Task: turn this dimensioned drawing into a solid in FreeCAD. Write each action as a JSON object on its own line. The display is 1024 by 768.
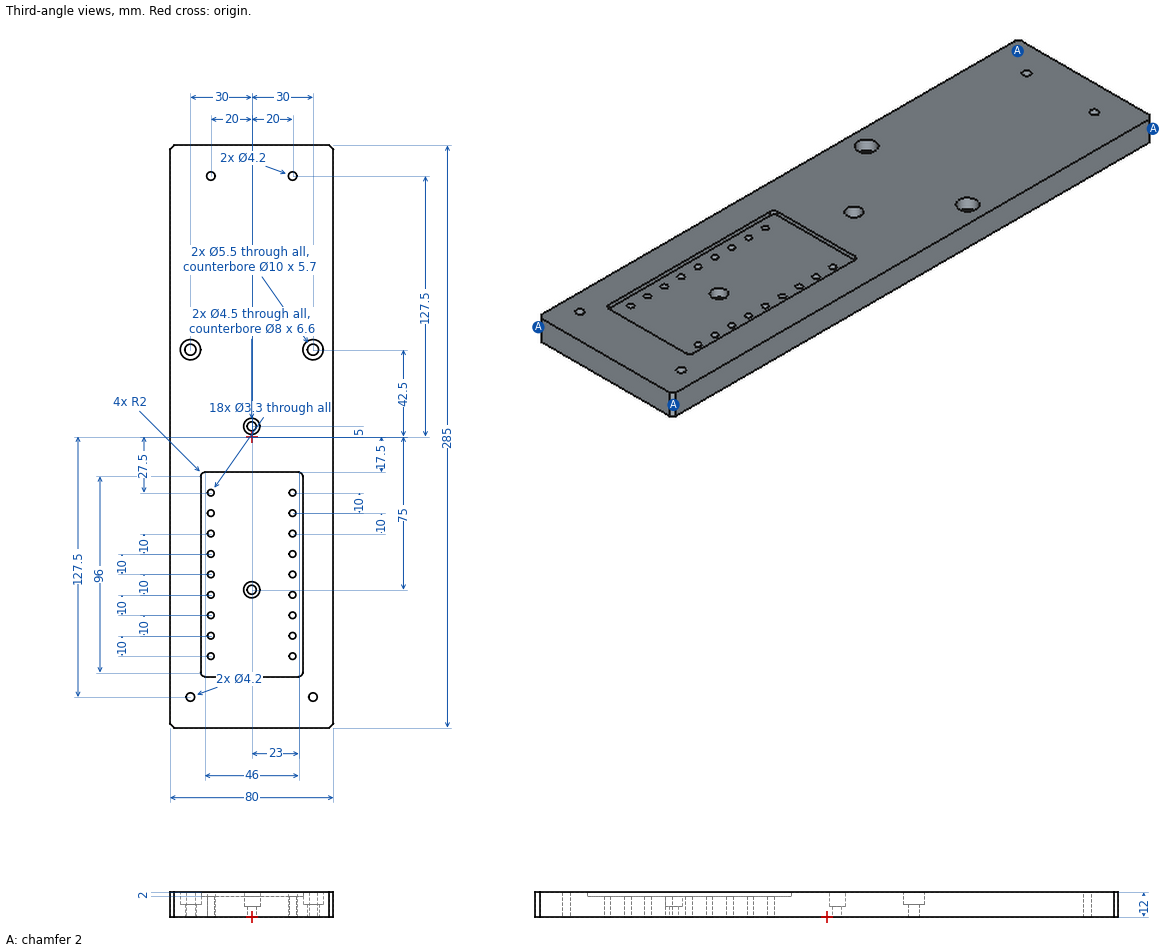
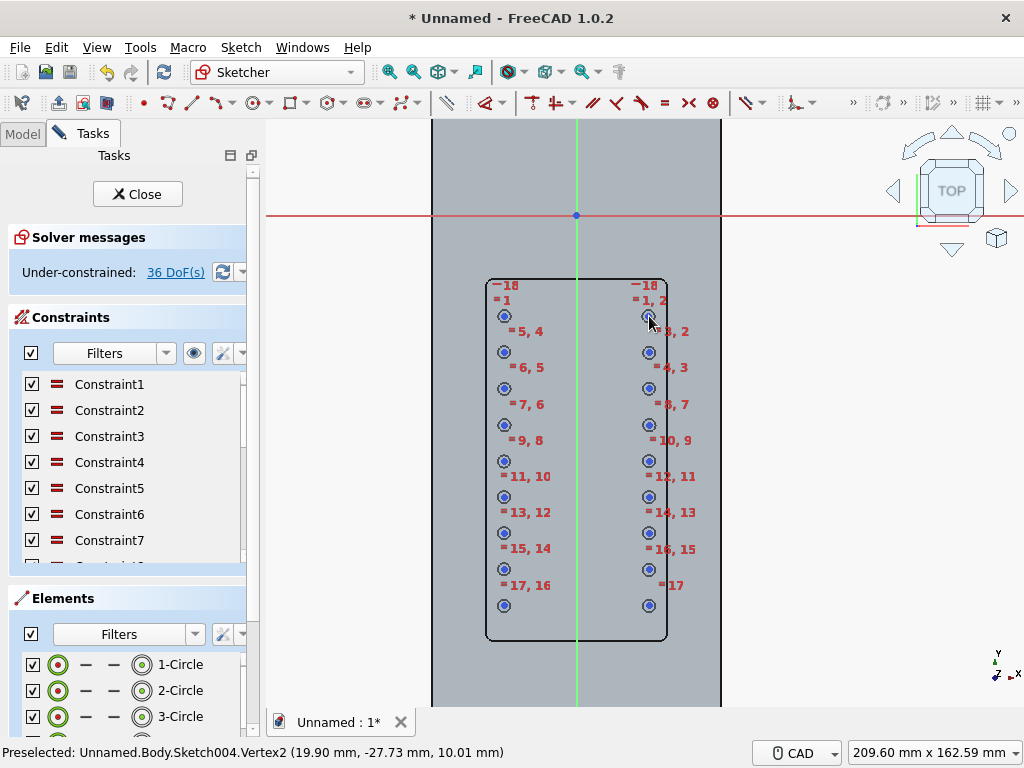
{"action": "left_click", "coordinate": [649, 316]}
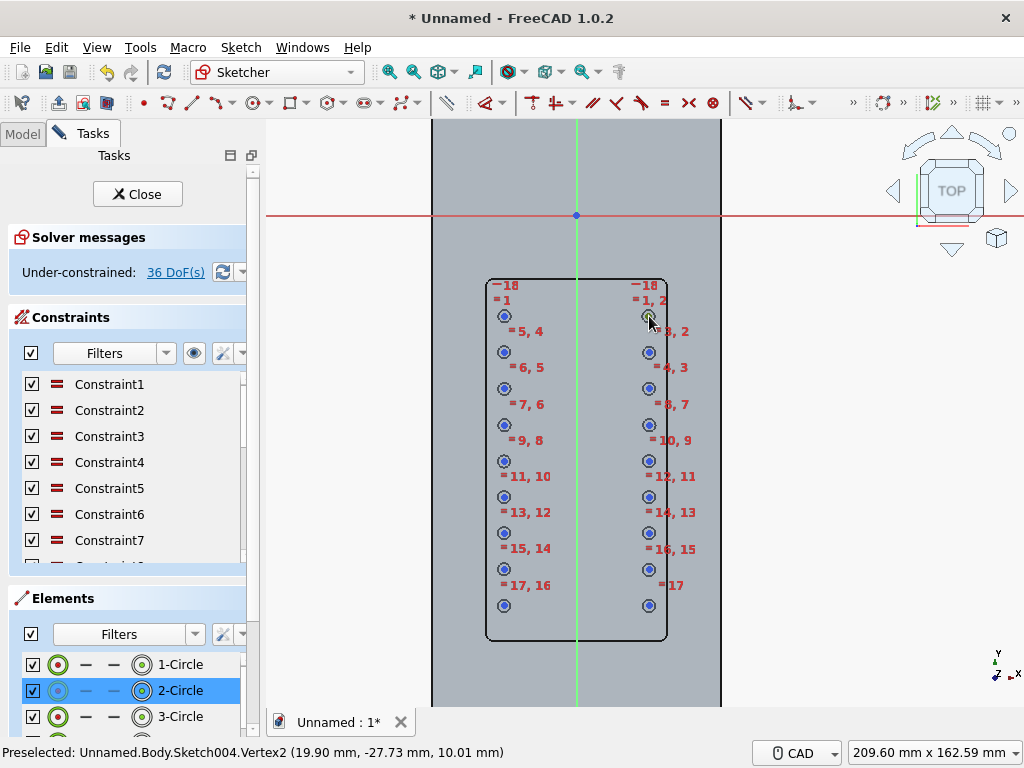
{"action": "left_click", "coordinate": [649, 353]}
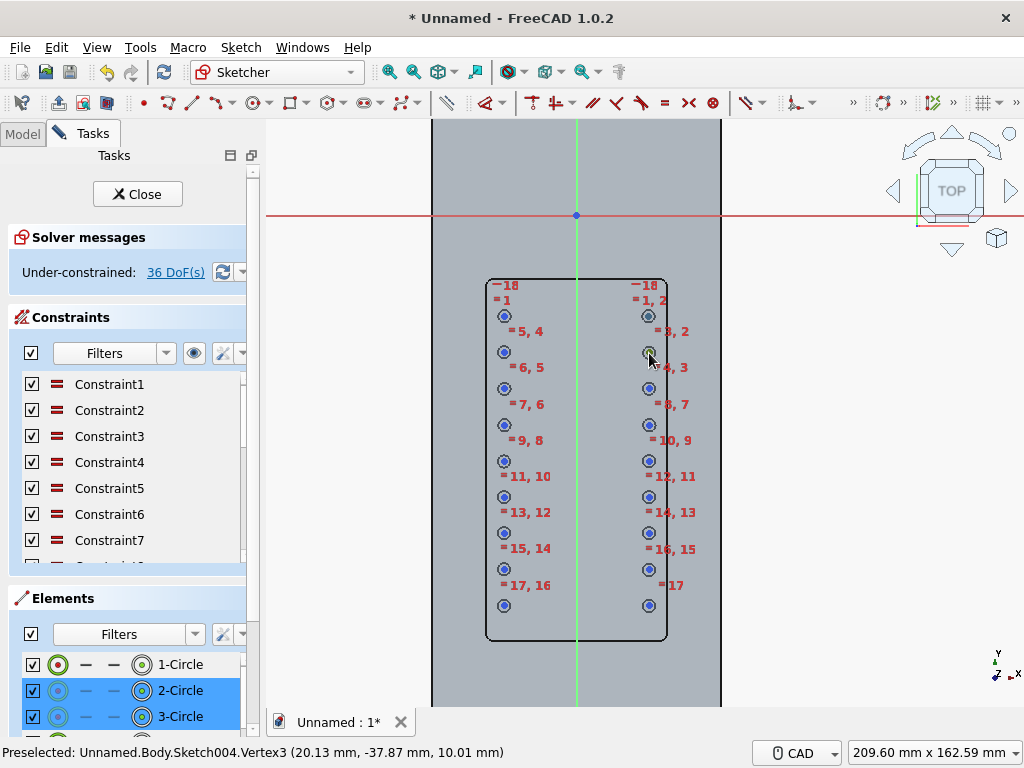
{"action": "key", "text": "v"}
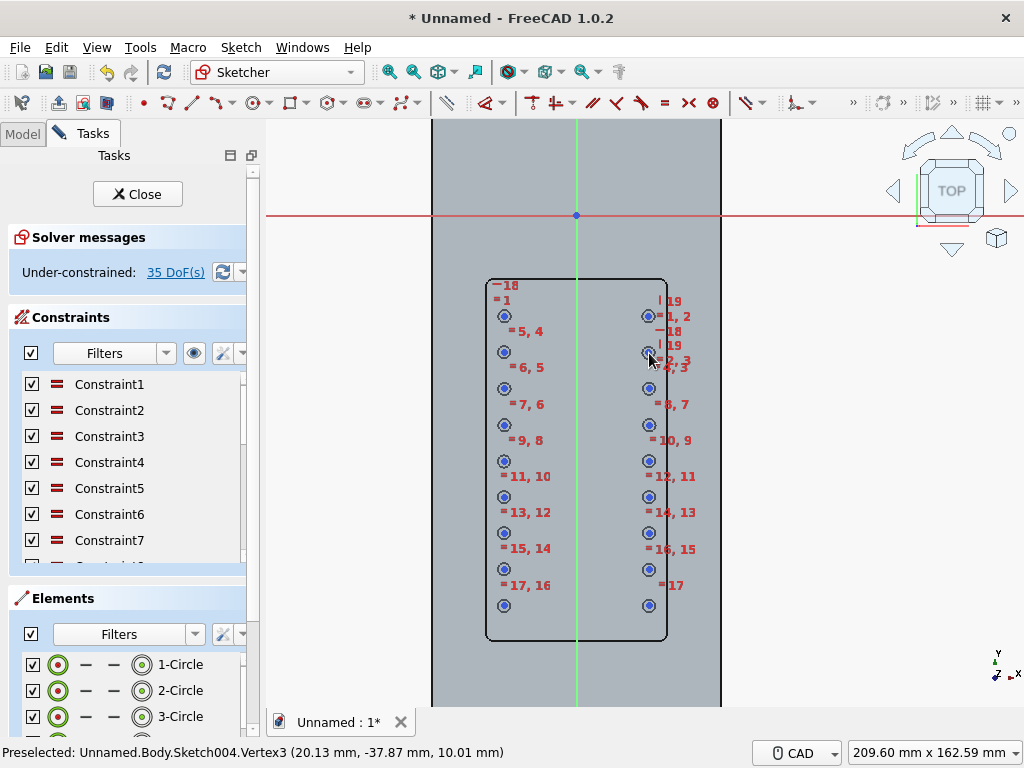
{"action": "left_click", "coordinate": [649, 353]}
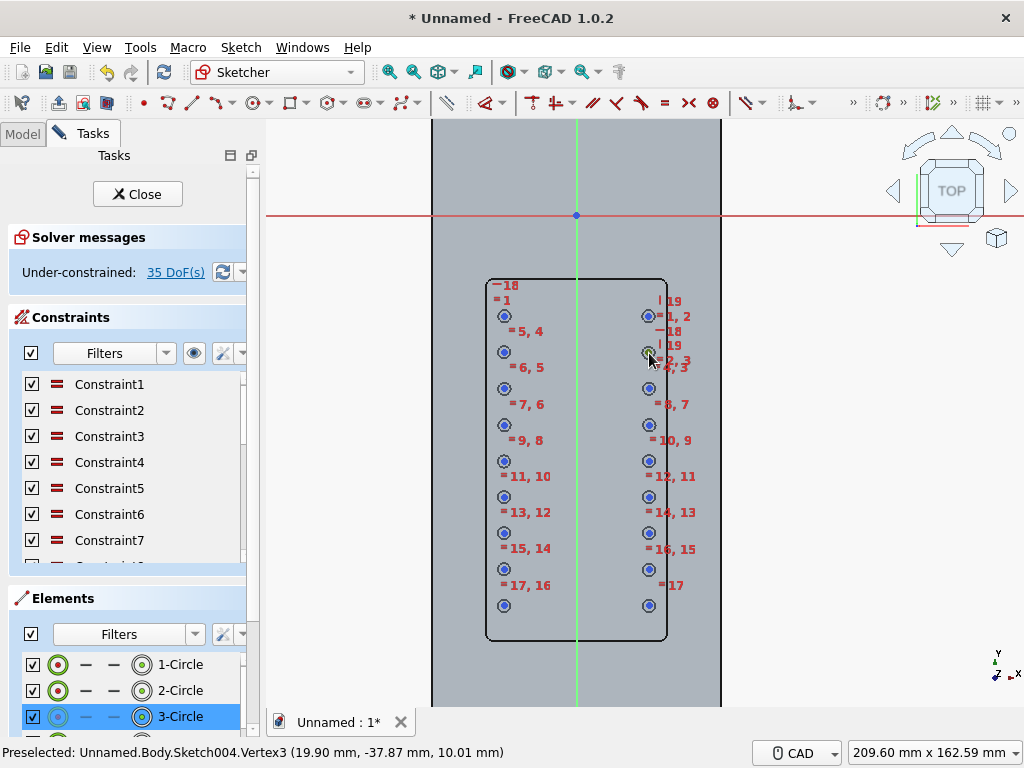
{"action": "left_click", "coordinate": [649, 389]}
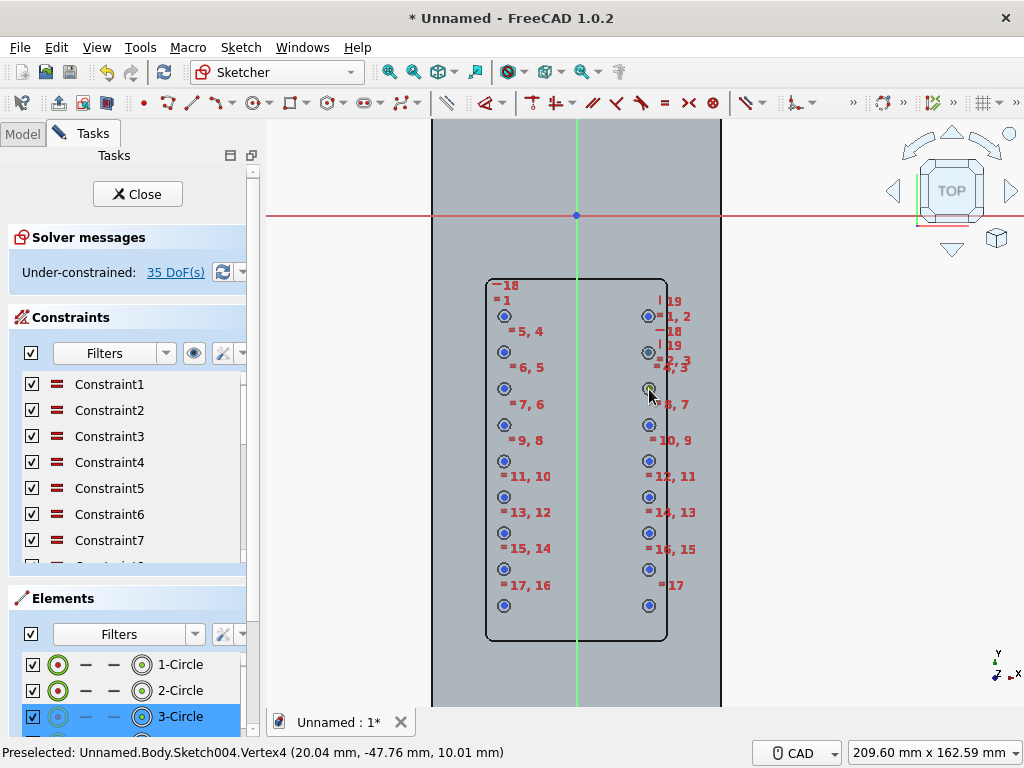
{"action": "key", "text": "v"}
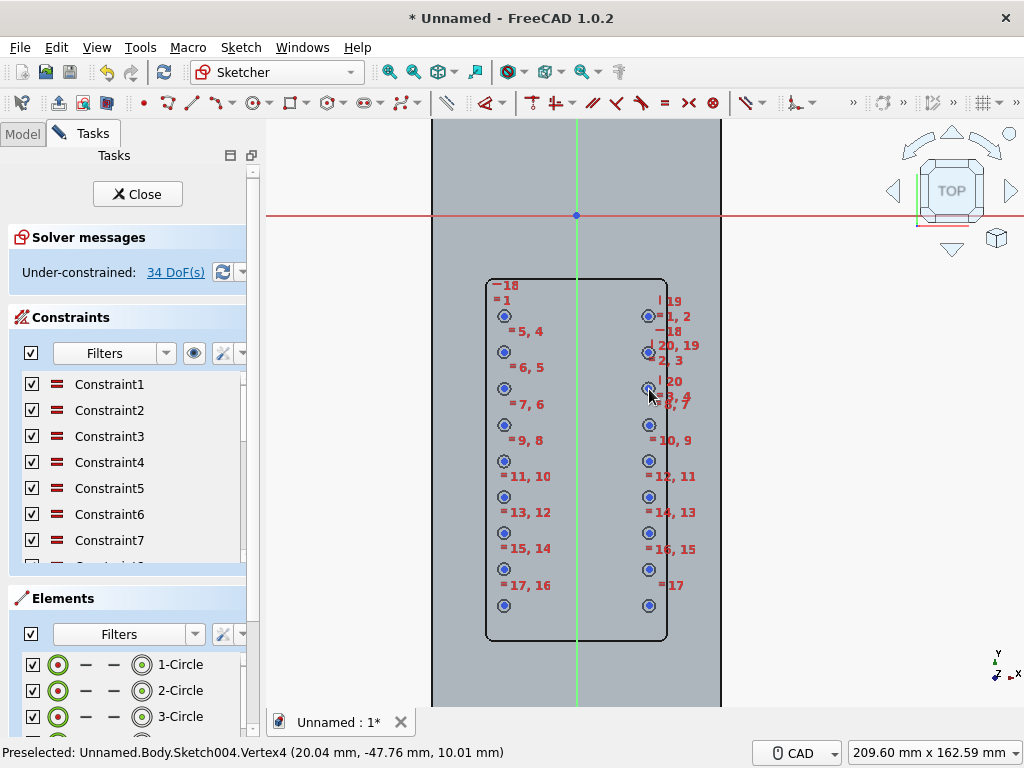
{"action": "left_click", "coordinate": [505, 316]}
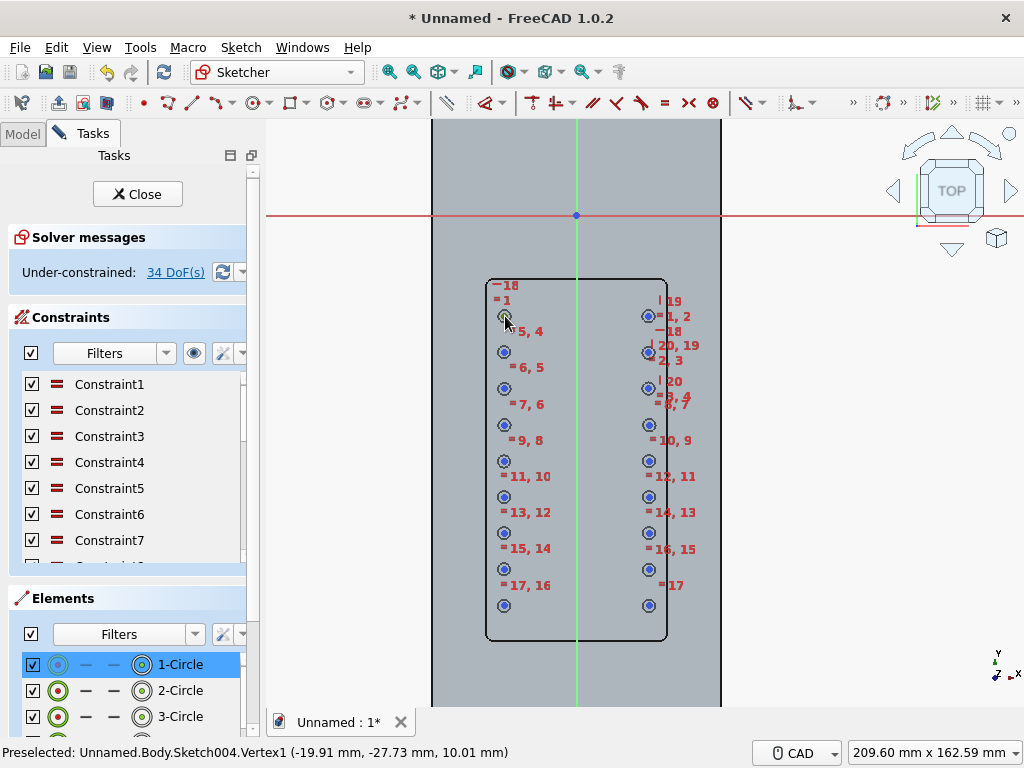
{"action": "left_click", "coordinate": [504, 352]}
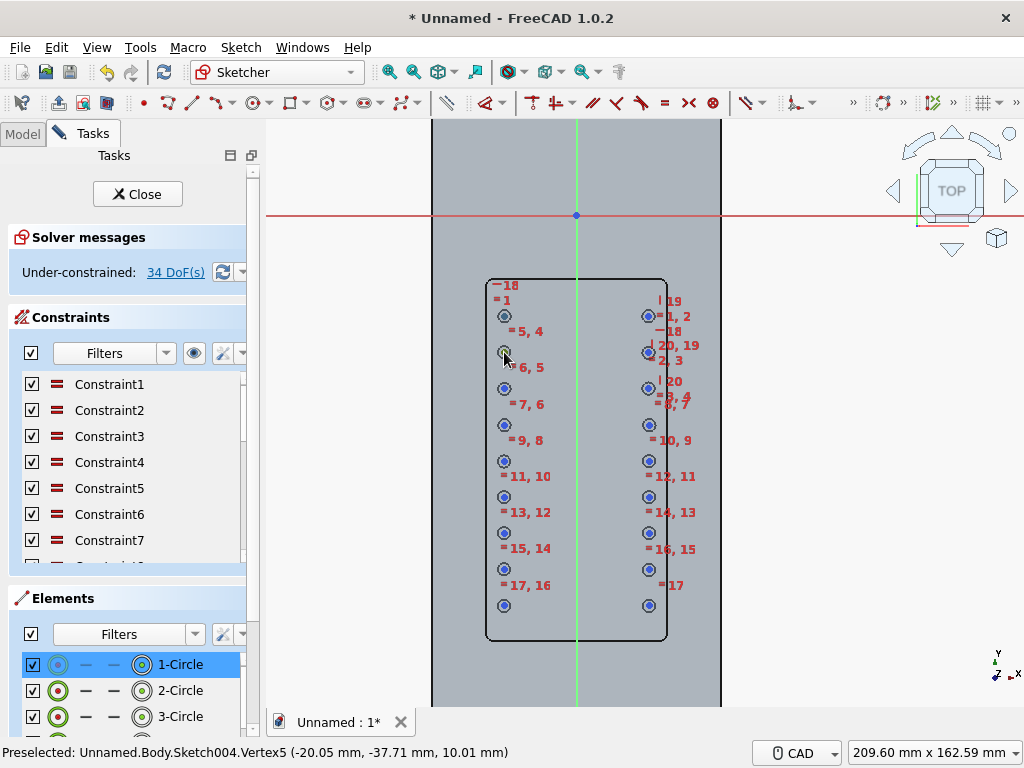
{"action": "key", "text": "v"}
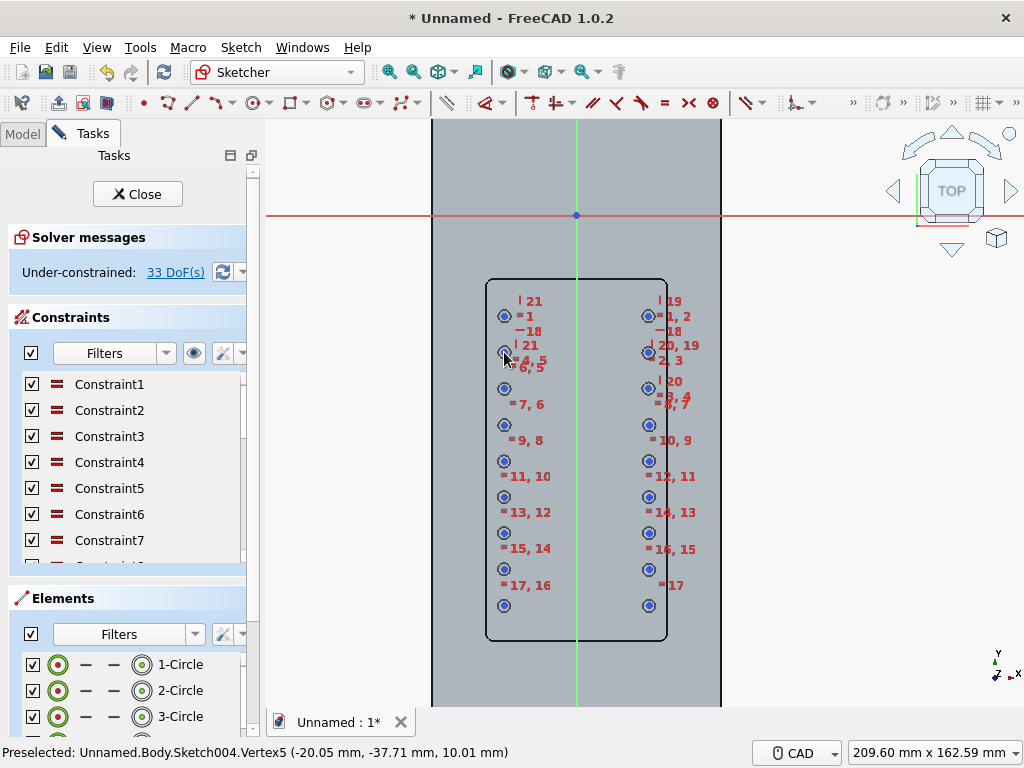
{"action": "left_click", "coordinate": [649, 353]}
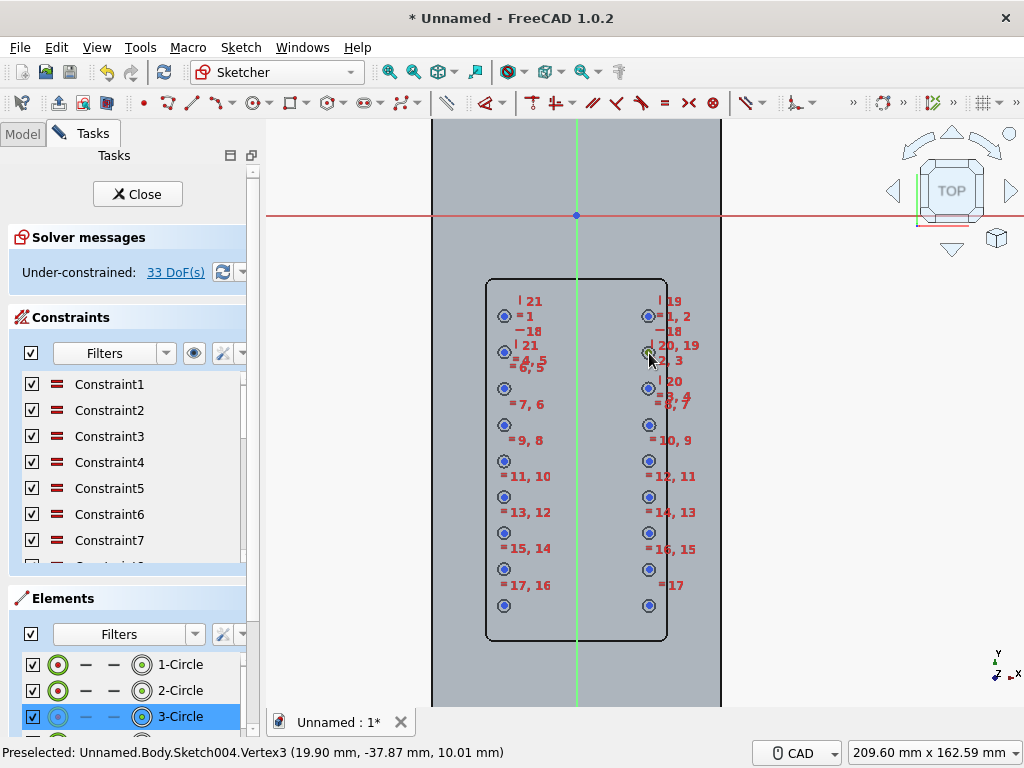
{"action": "left_click", "coordinate": [505, 352]}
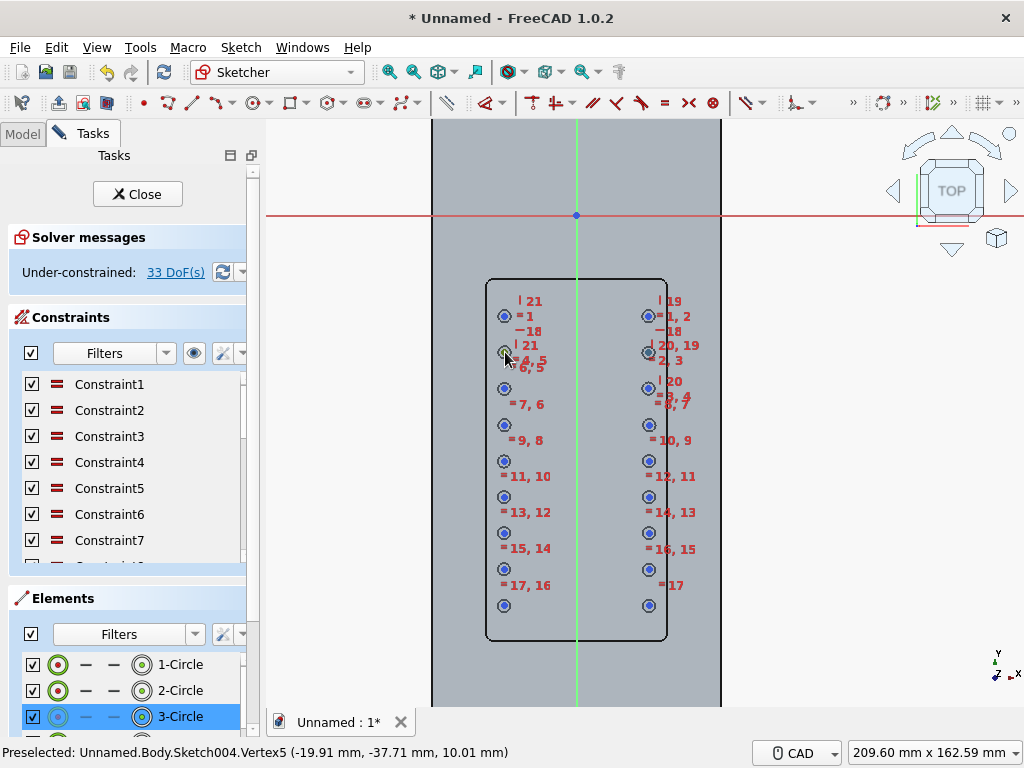
{"action": "key", "text": "h"}